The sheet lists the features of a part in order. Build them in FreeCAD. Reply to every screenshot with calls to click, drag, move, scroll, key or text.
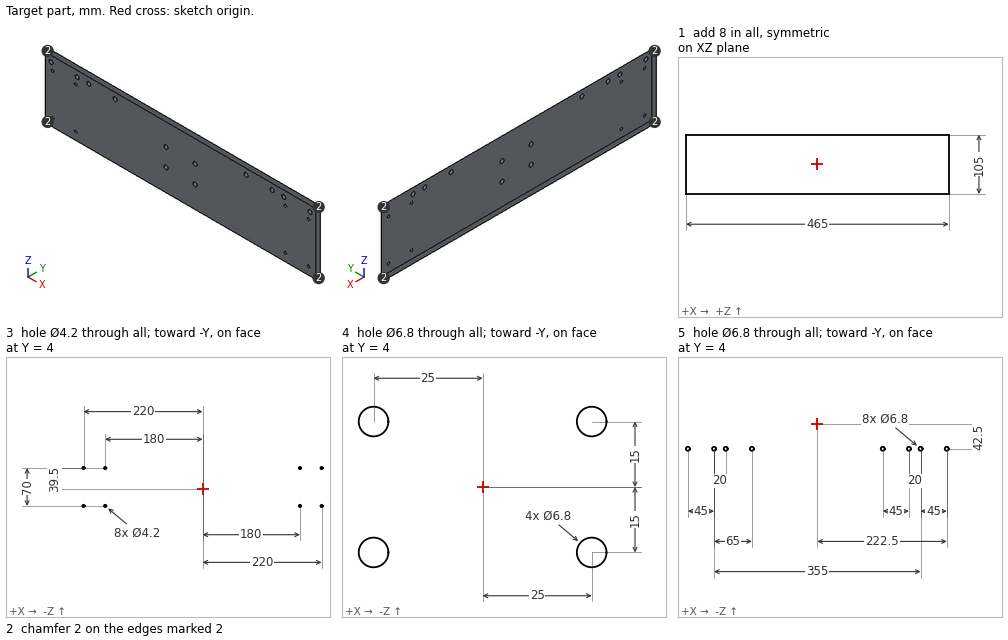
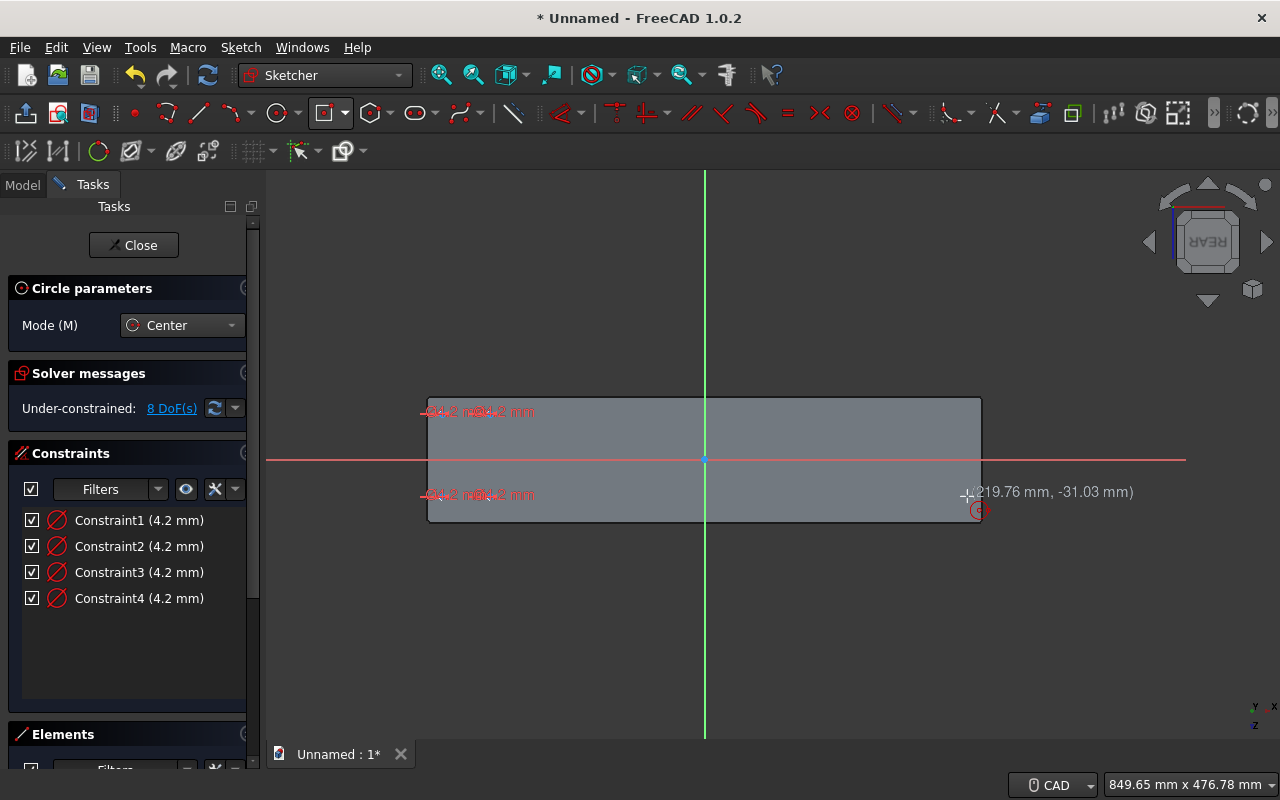
click(967, 496)
move(969, 495)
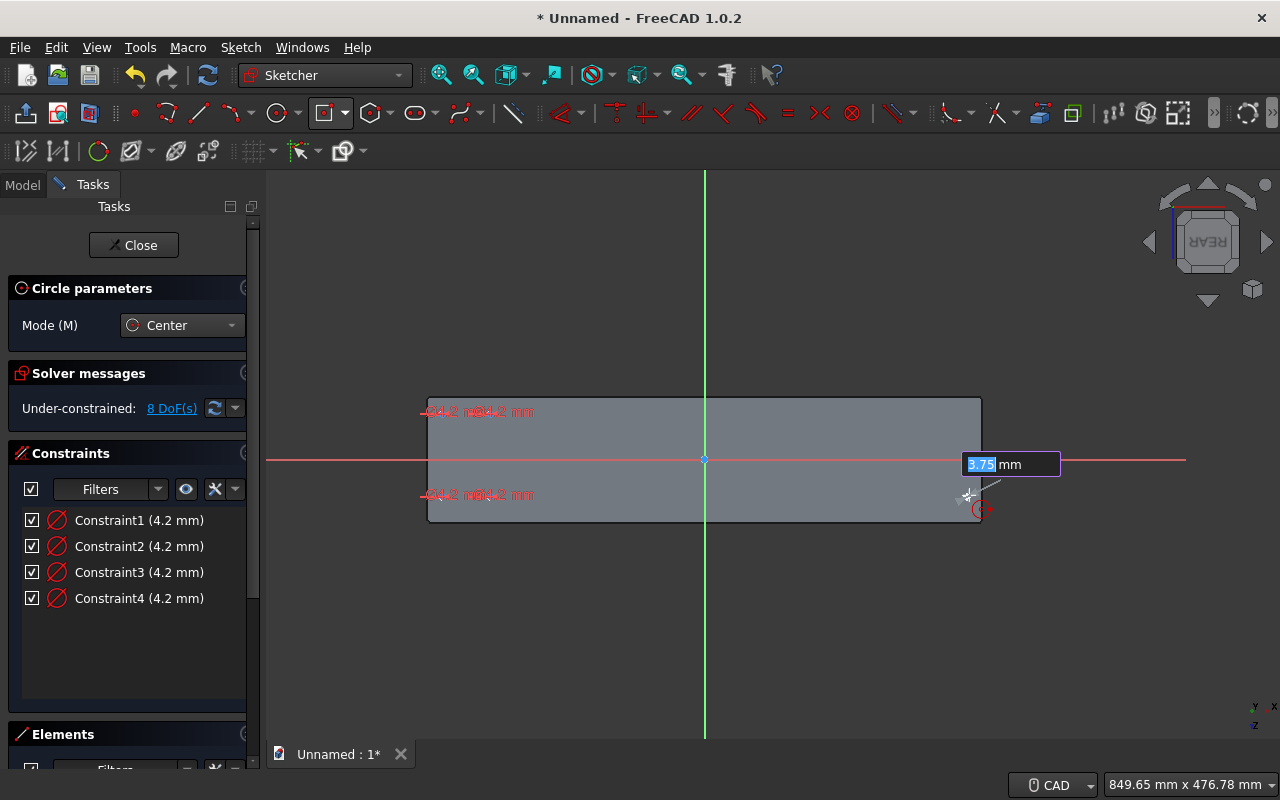
text(4.2)
key(Return)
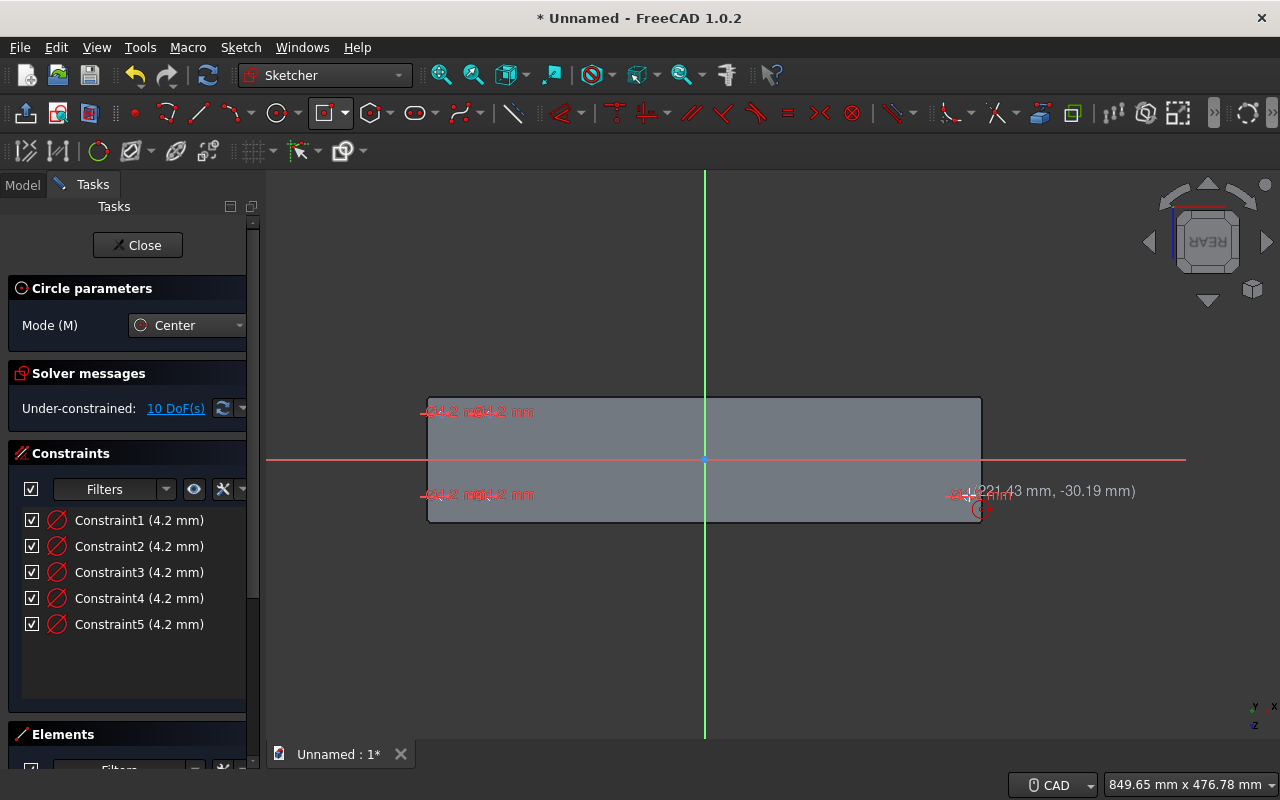
scroll(920, 496, up, 12)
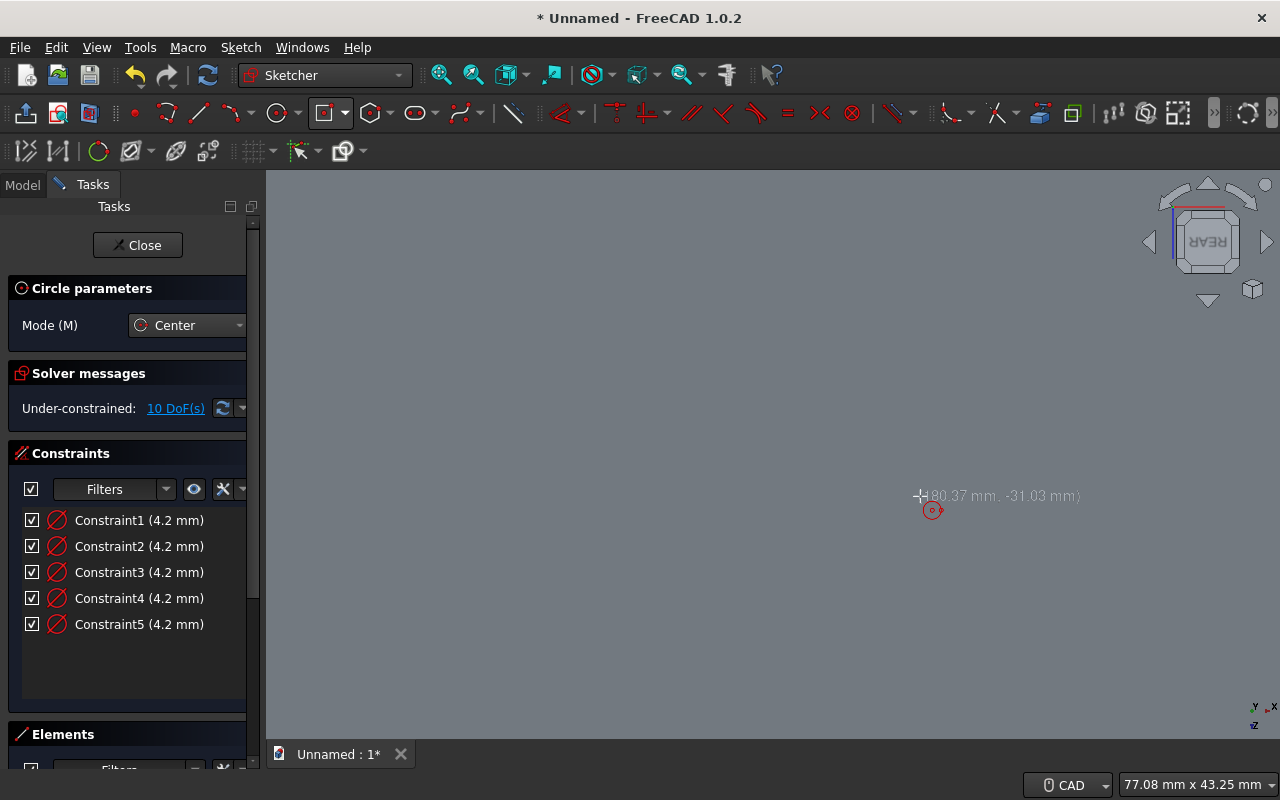
scroll(920, 496, down, 12)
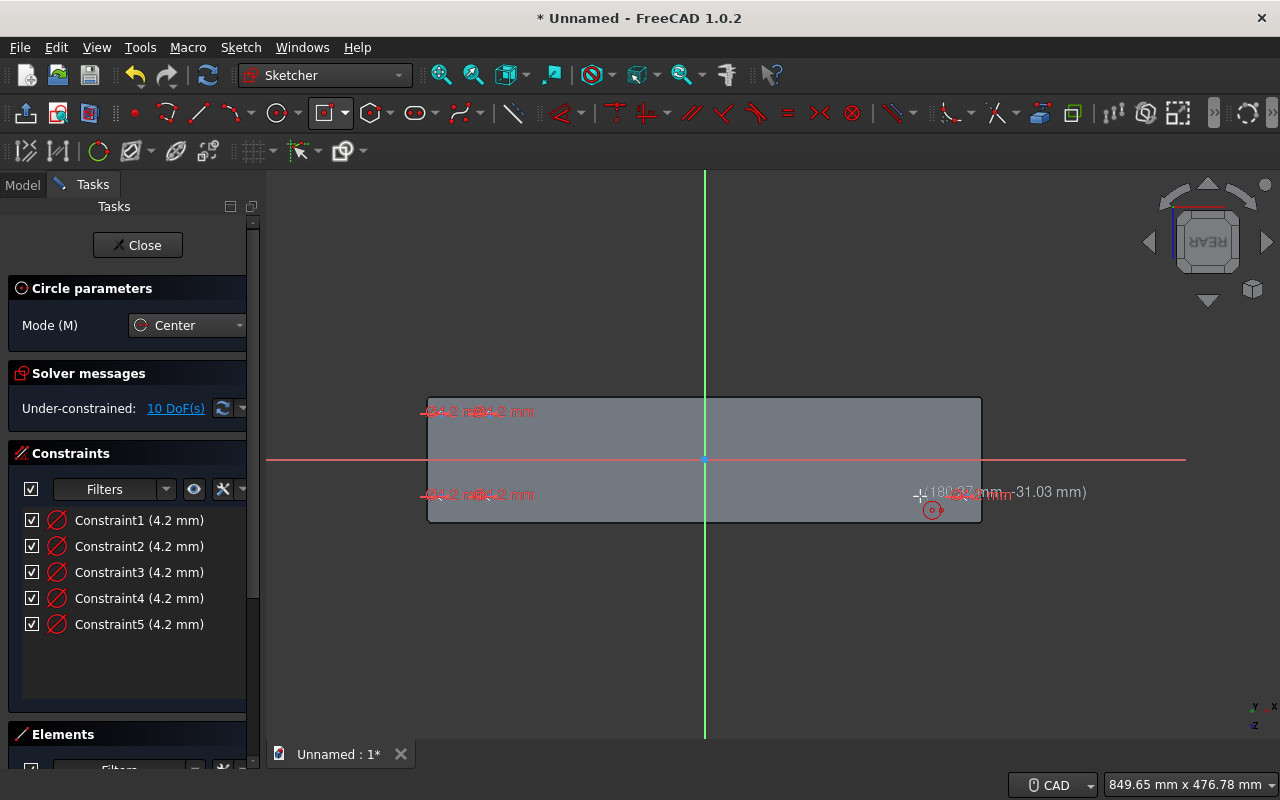
click(920, 496)
move(921, 495)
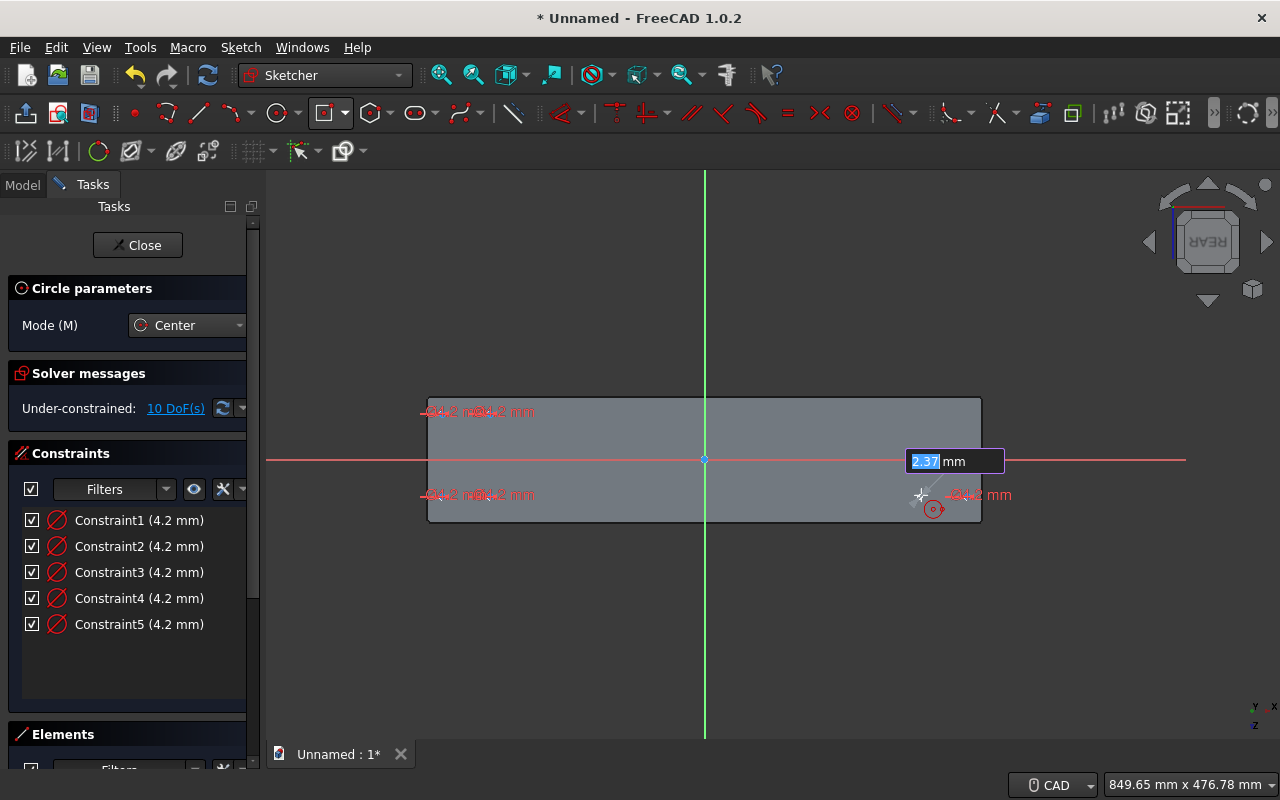
text(4.2)
key(Return)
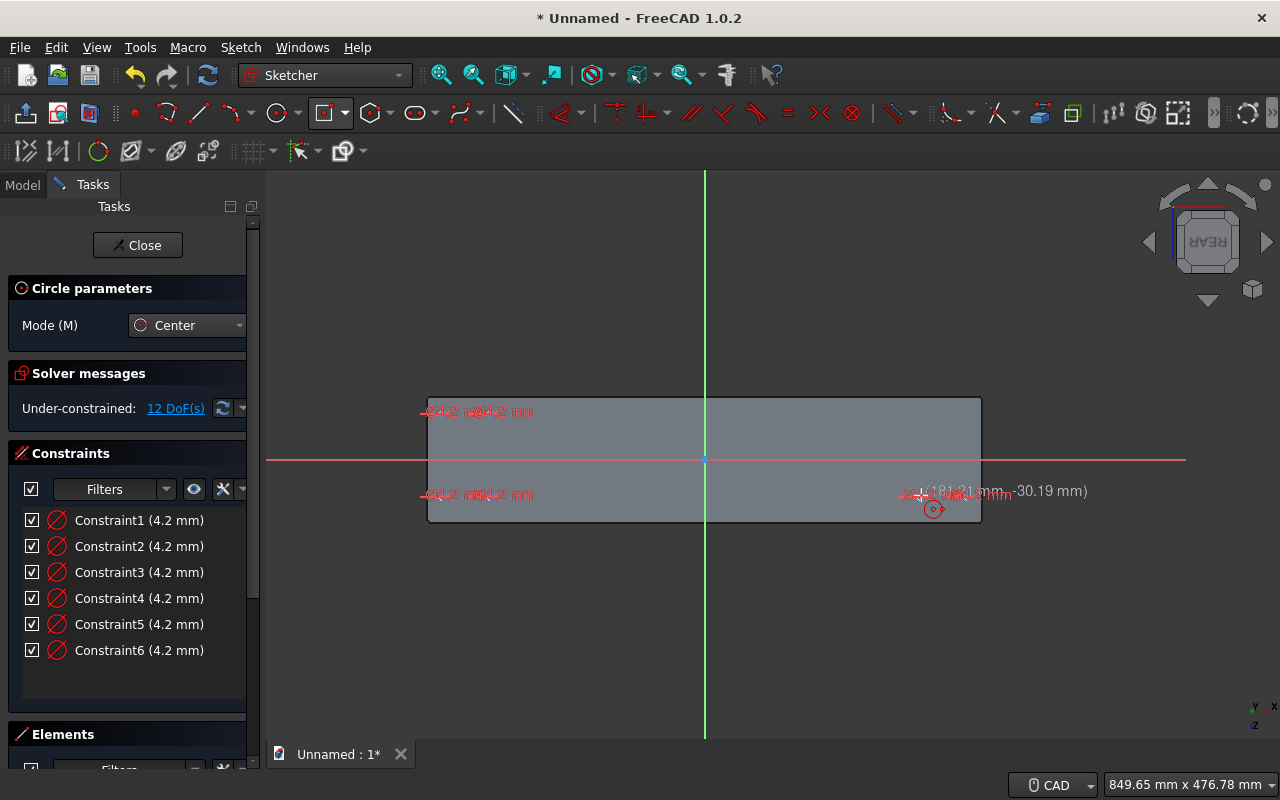
scroll(920, 413, up, 12)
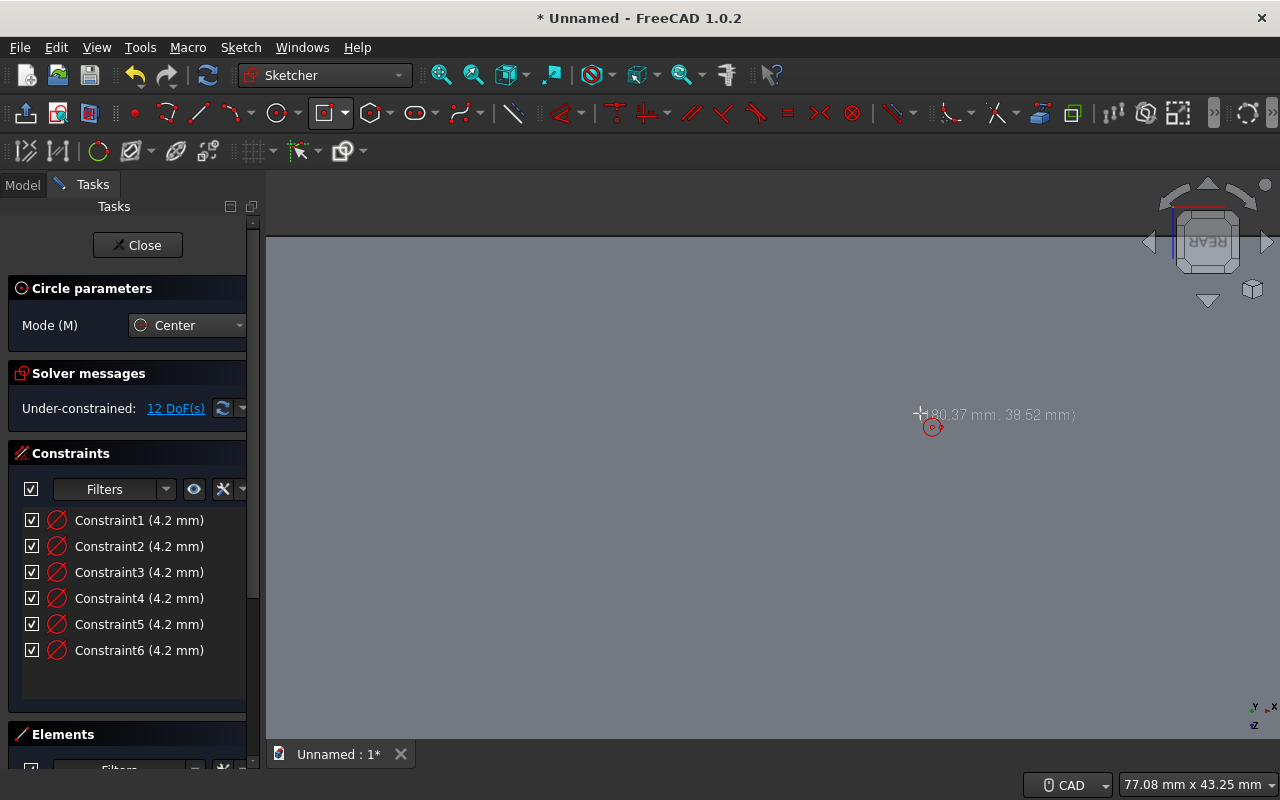
scroll(920, 413, down, 12)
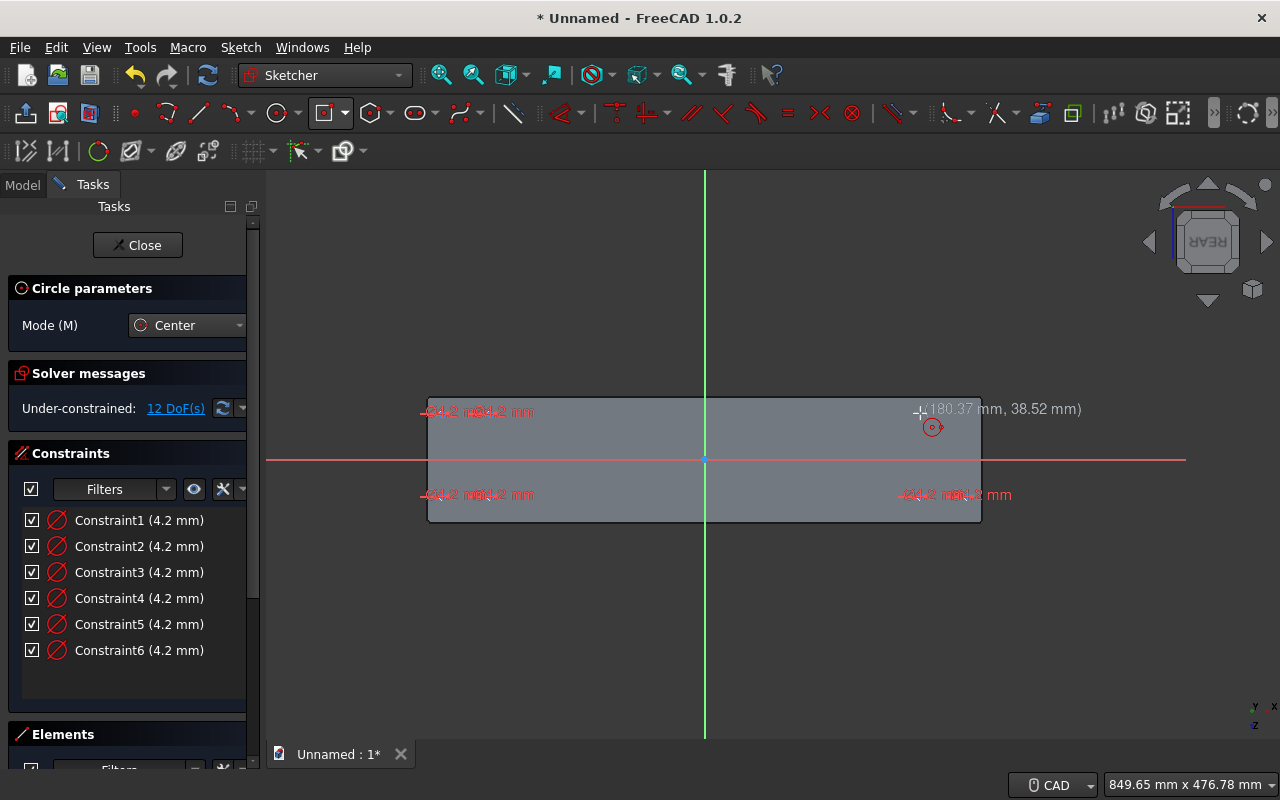
click(920, 413)
move(921, 411)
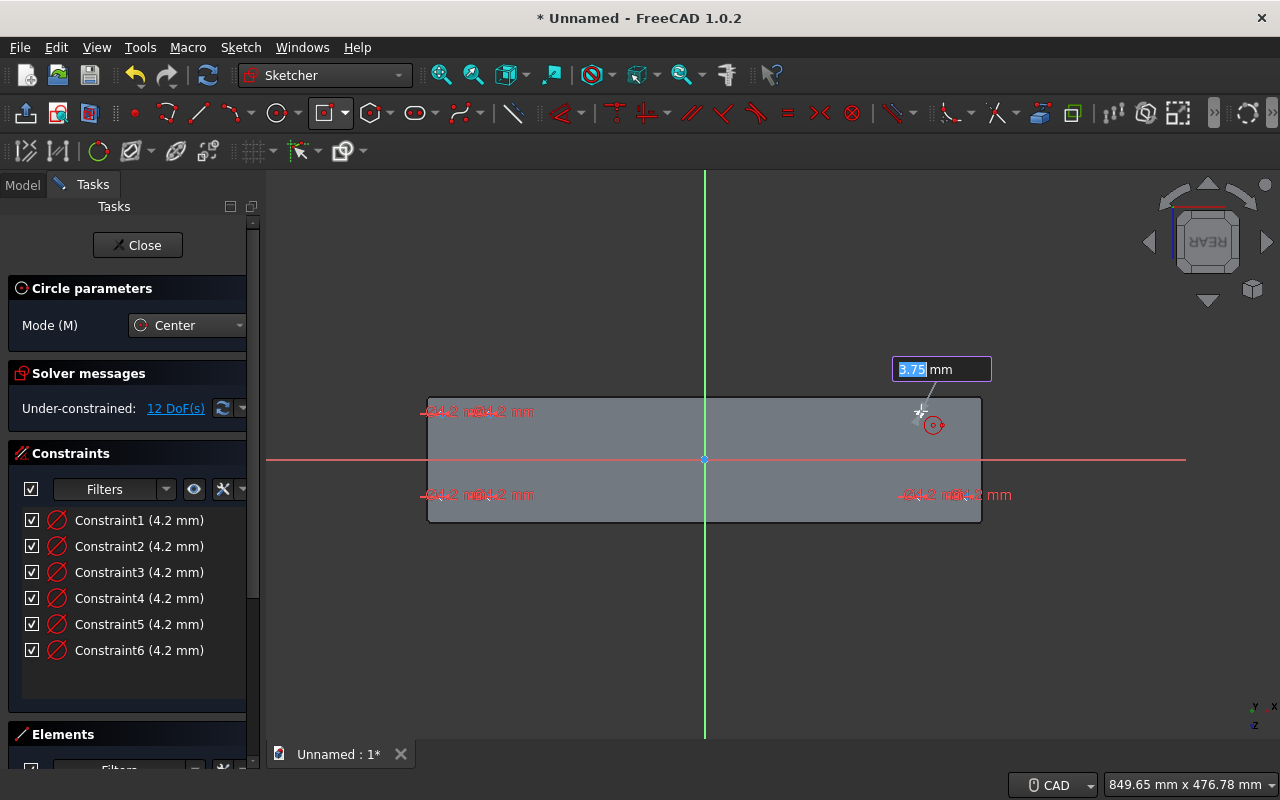
text(4.2)
key(Return)